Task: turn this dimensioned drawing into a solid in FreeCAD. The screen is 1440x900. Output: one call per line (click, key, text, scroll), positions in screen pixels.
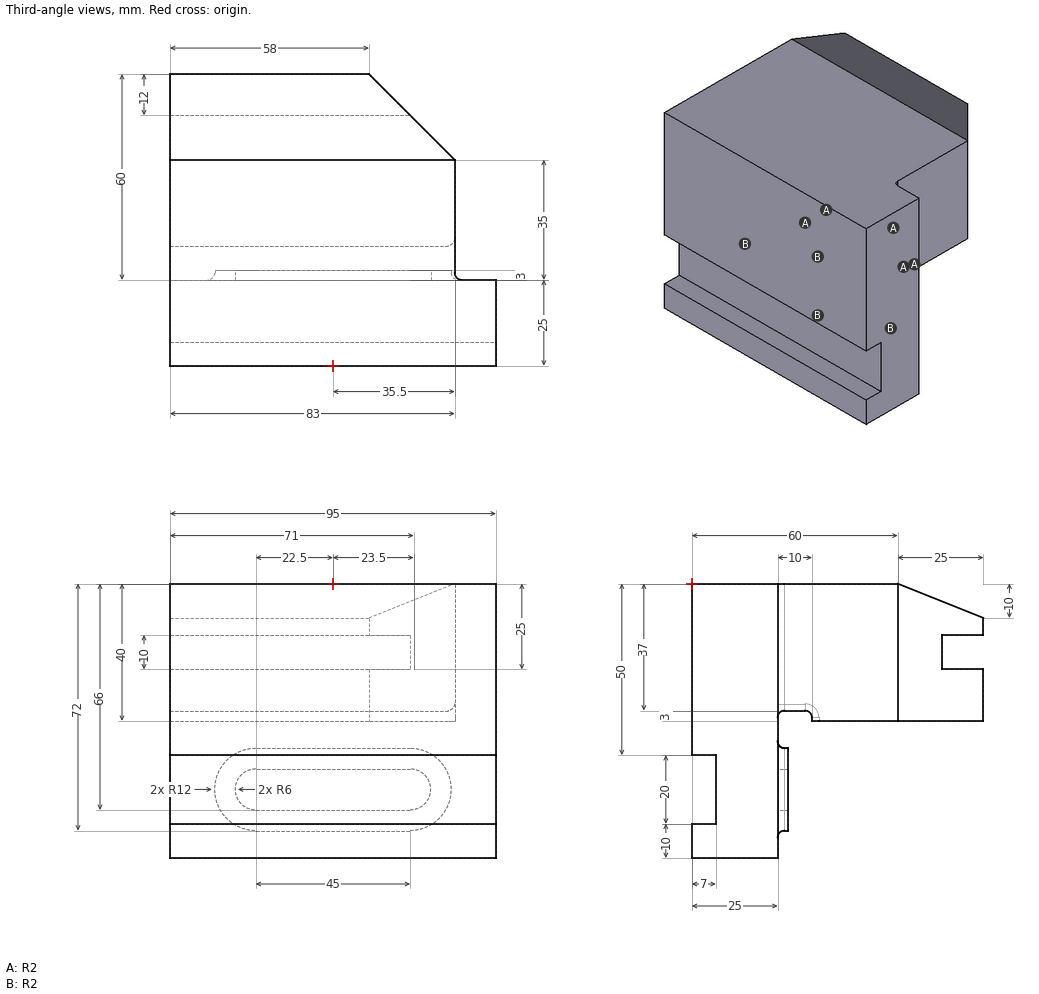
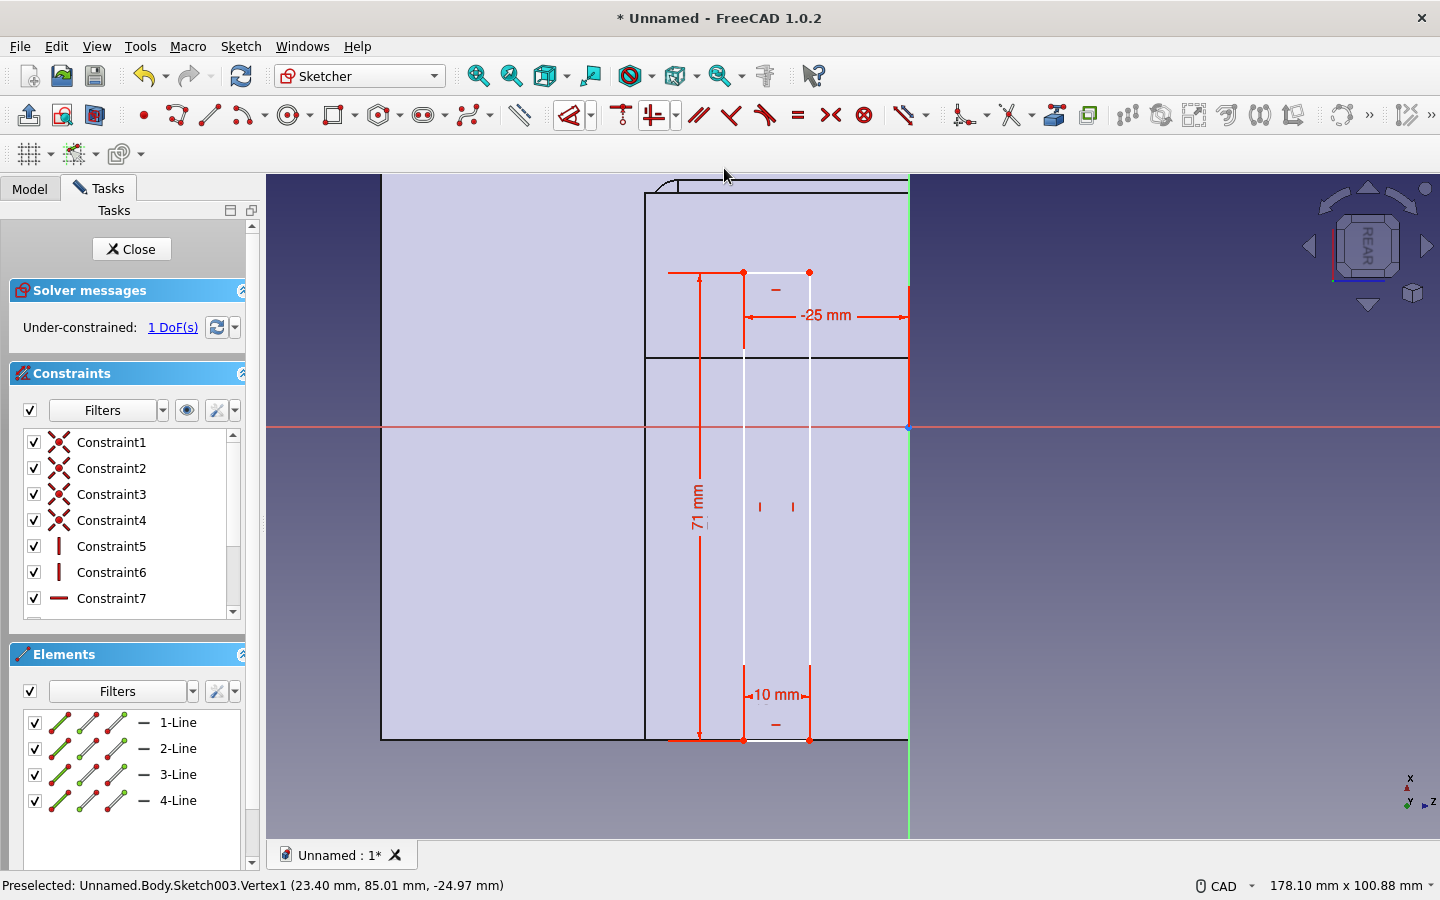
click(744, 273)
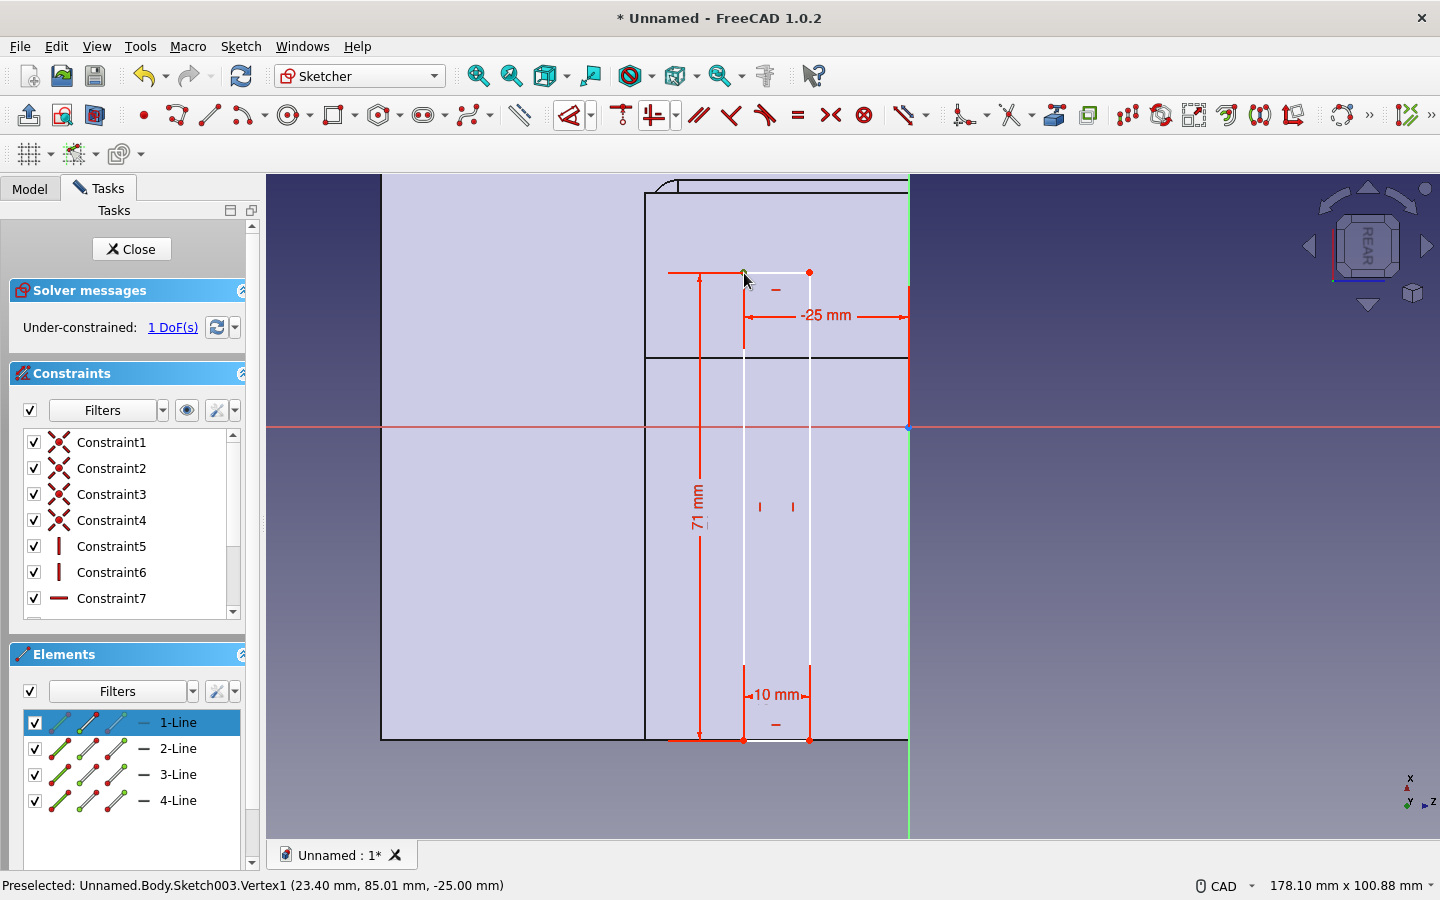
key(i)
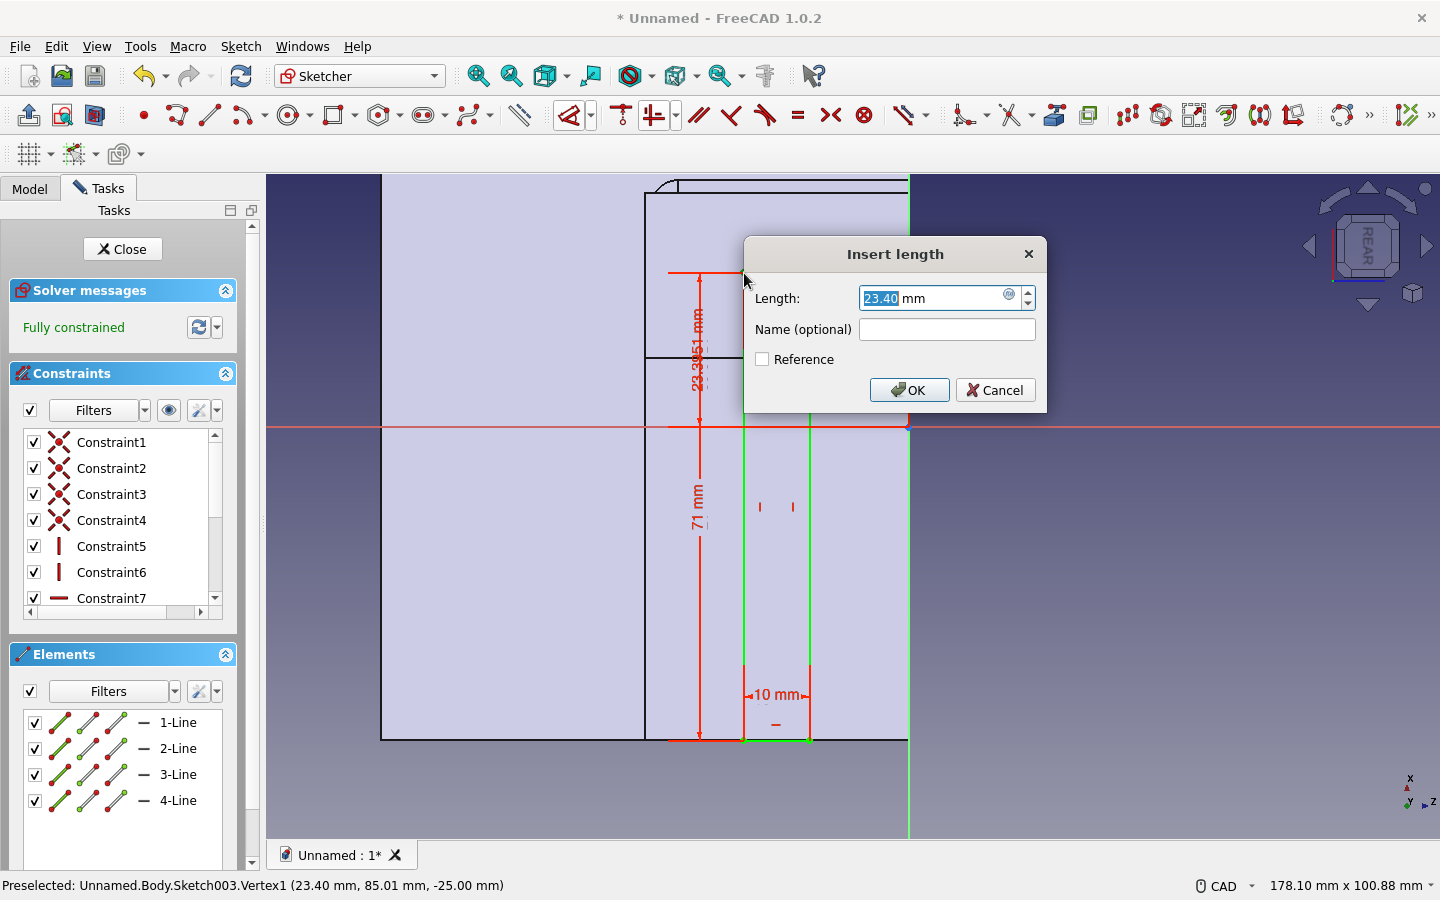
text(23.5)
key(Return)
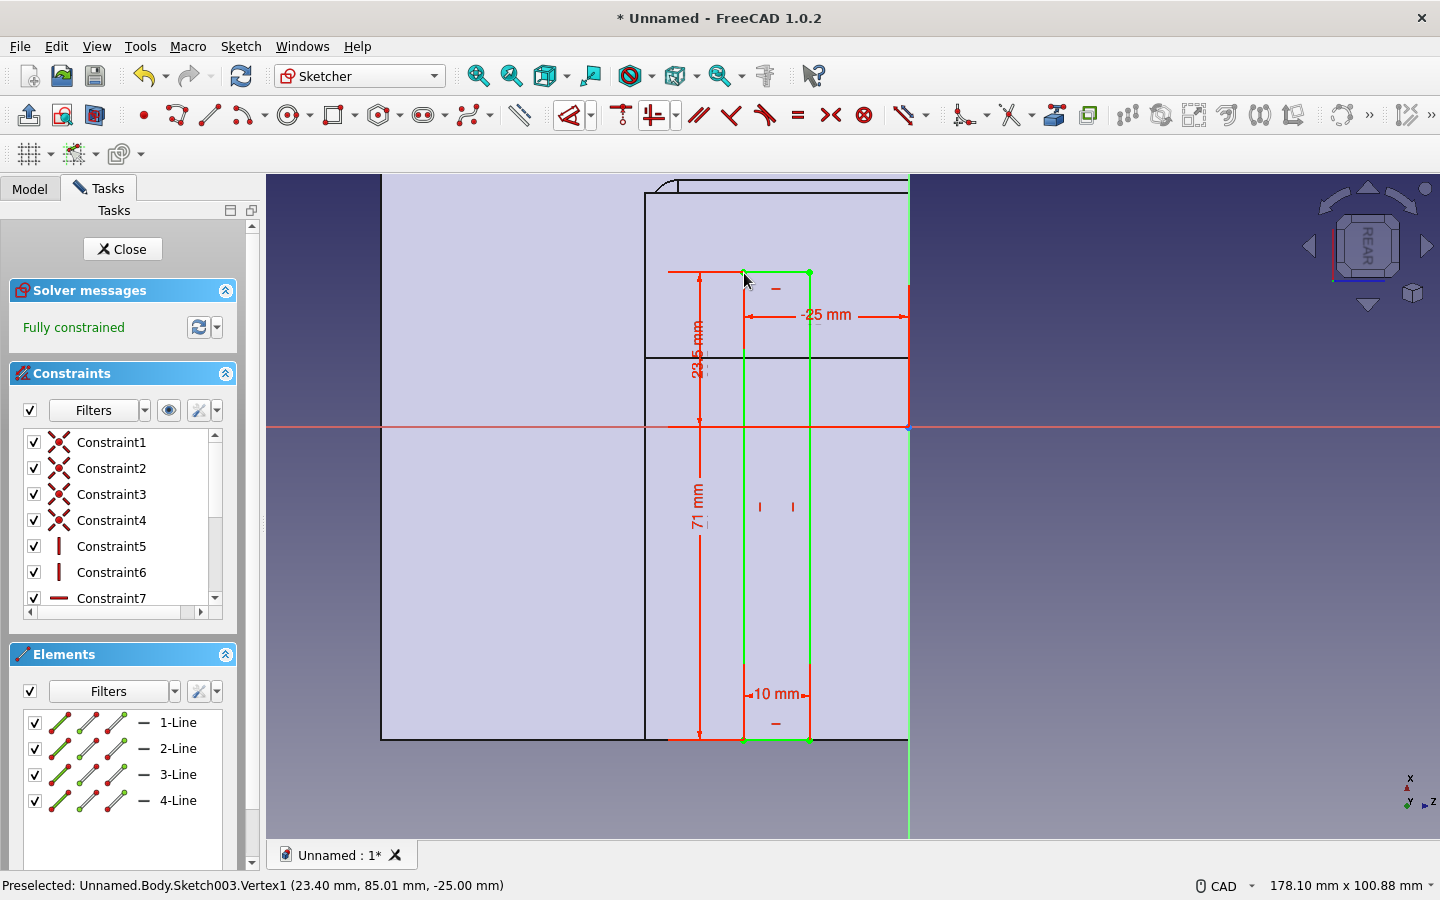
click(123, 249)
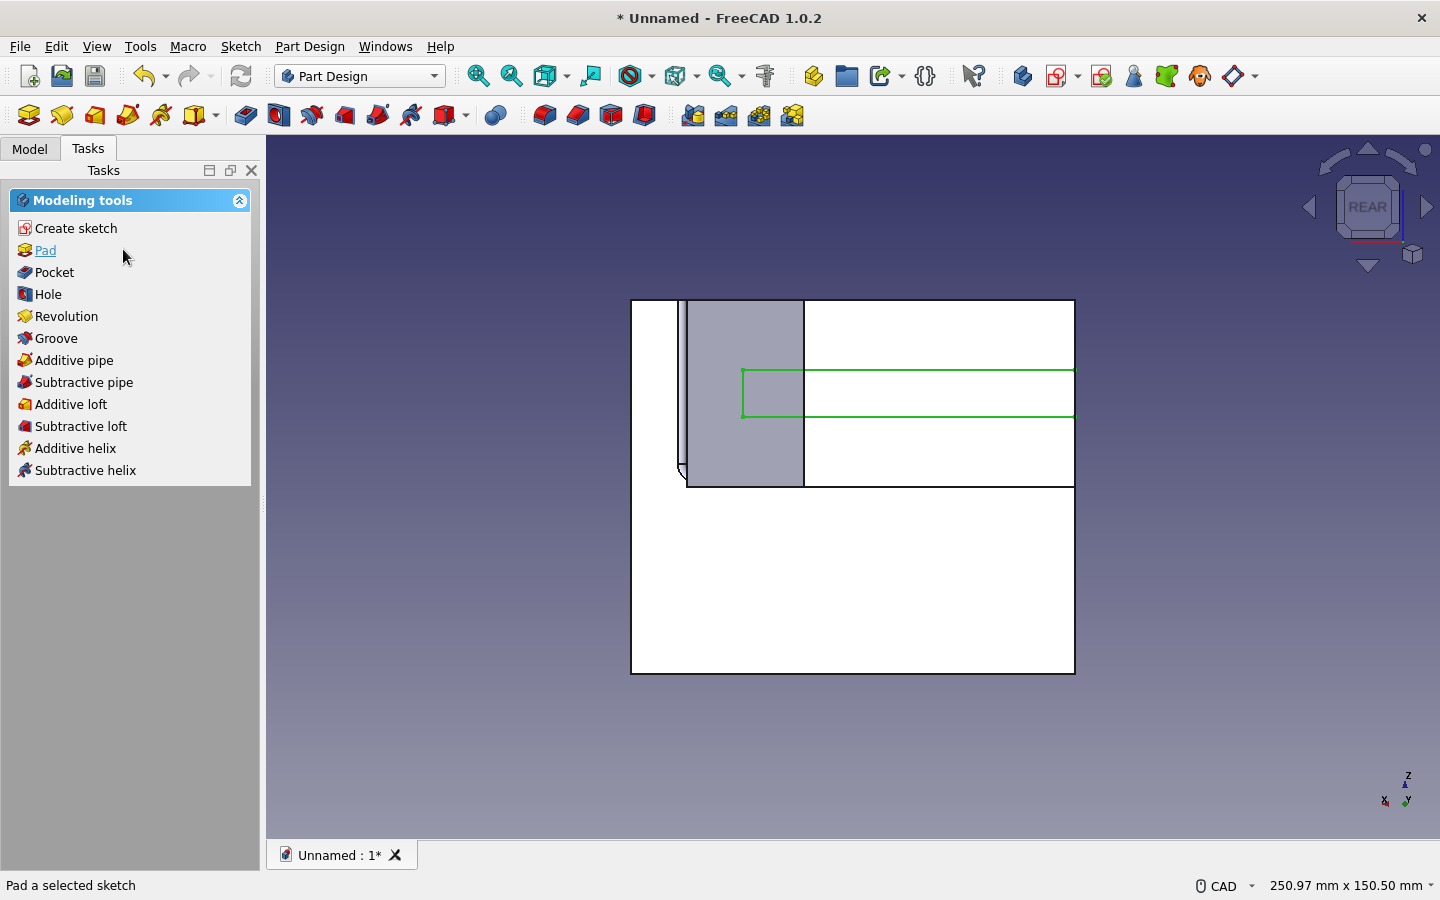
click(246, 116)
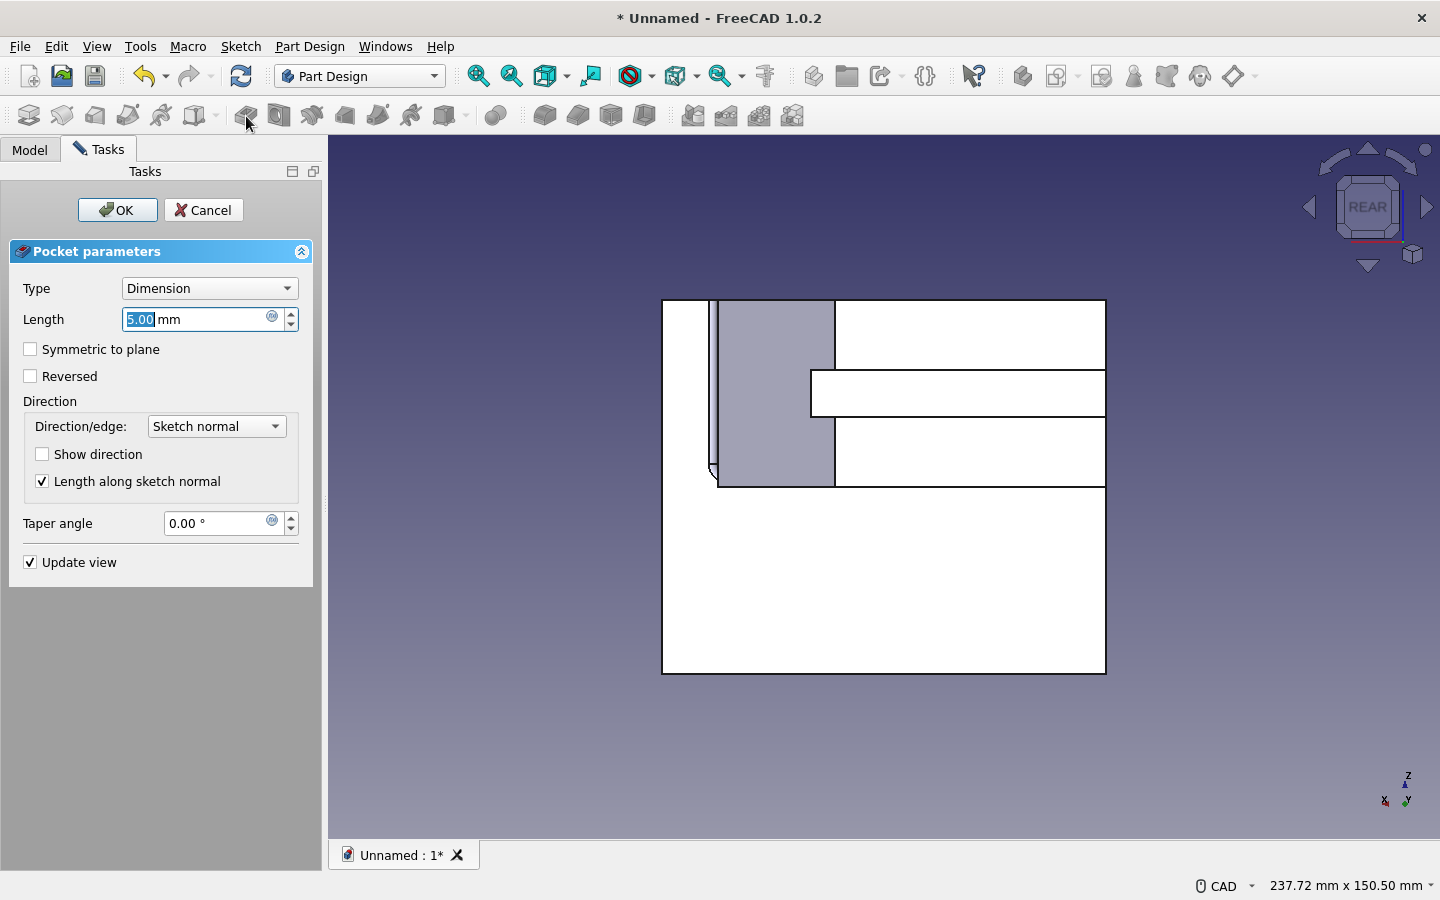
text(12)
key(Tab)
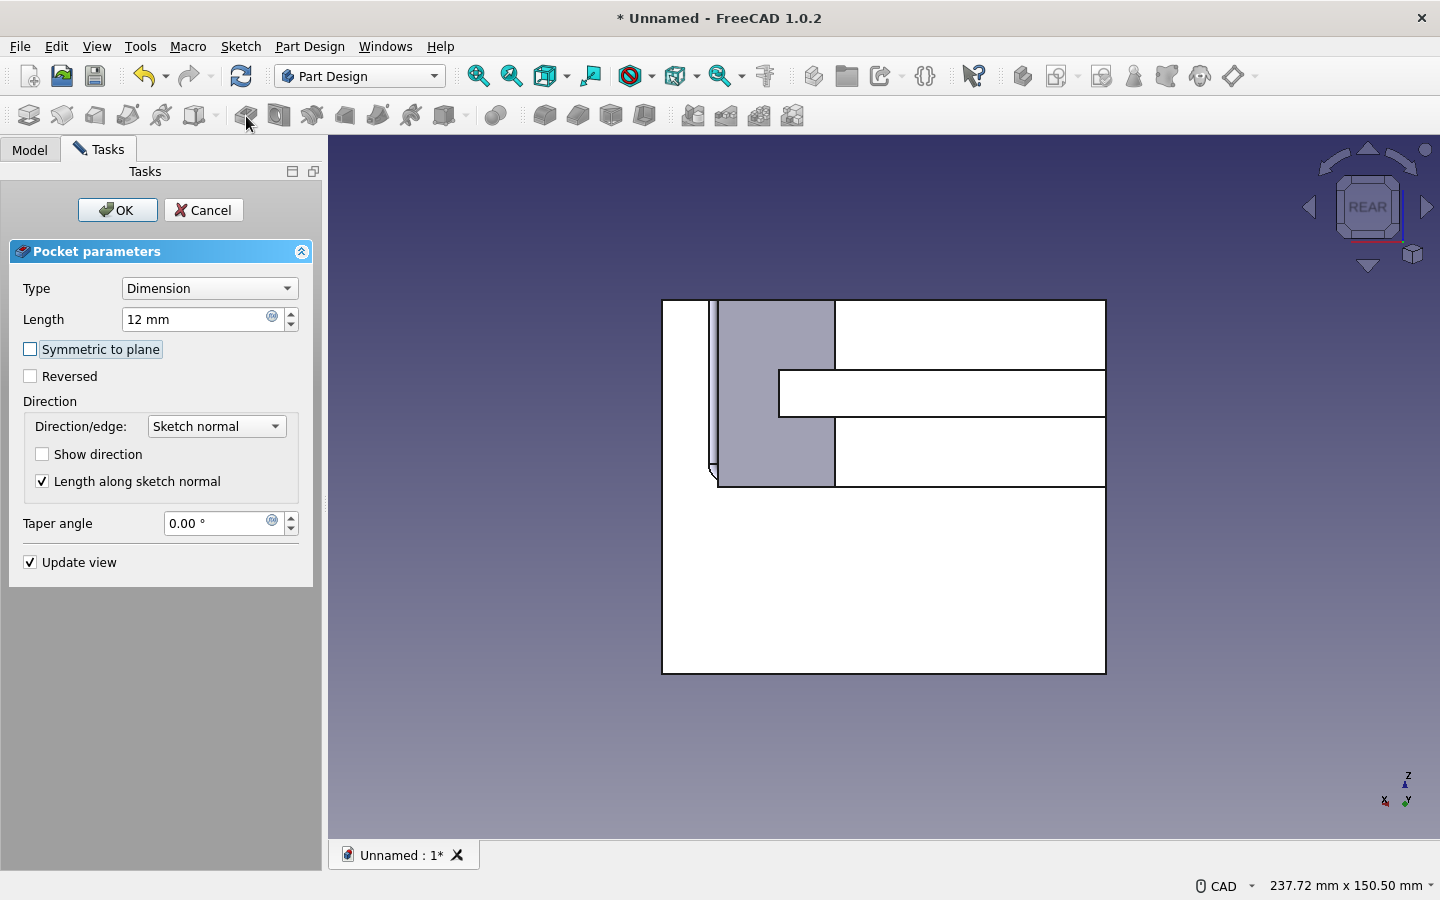
click(118, 210)